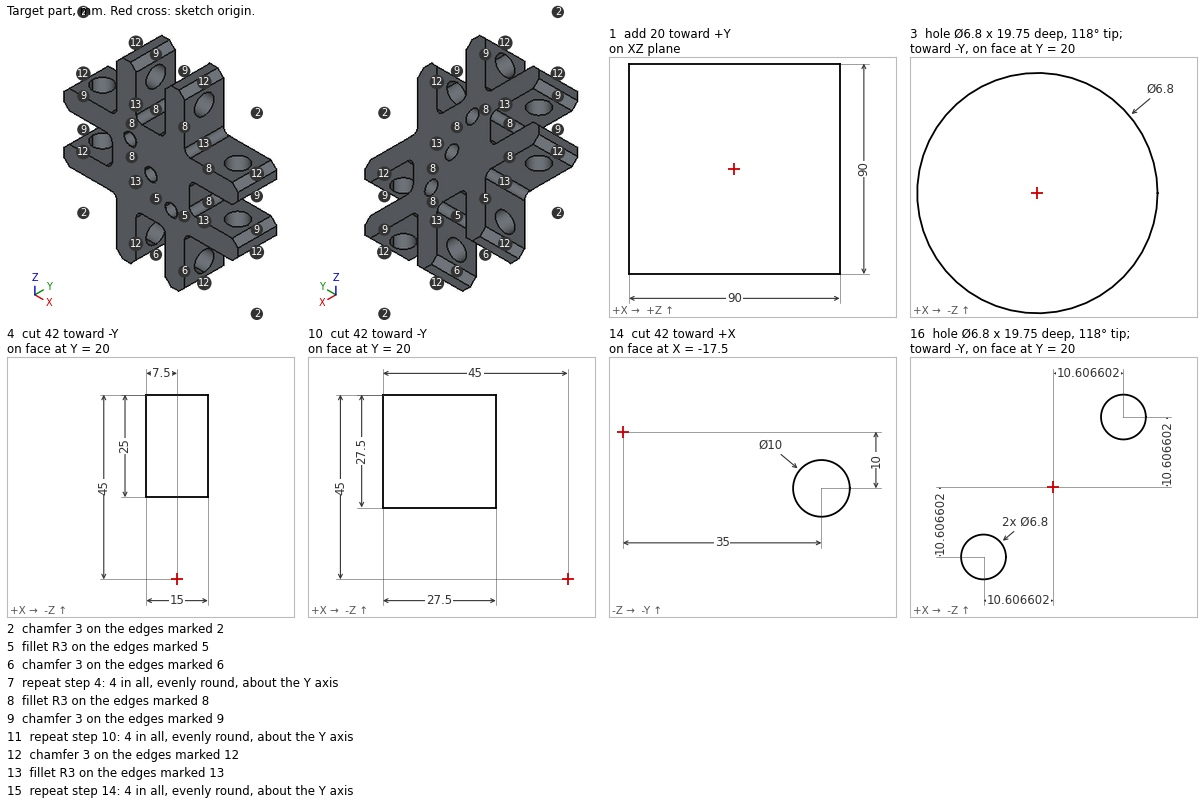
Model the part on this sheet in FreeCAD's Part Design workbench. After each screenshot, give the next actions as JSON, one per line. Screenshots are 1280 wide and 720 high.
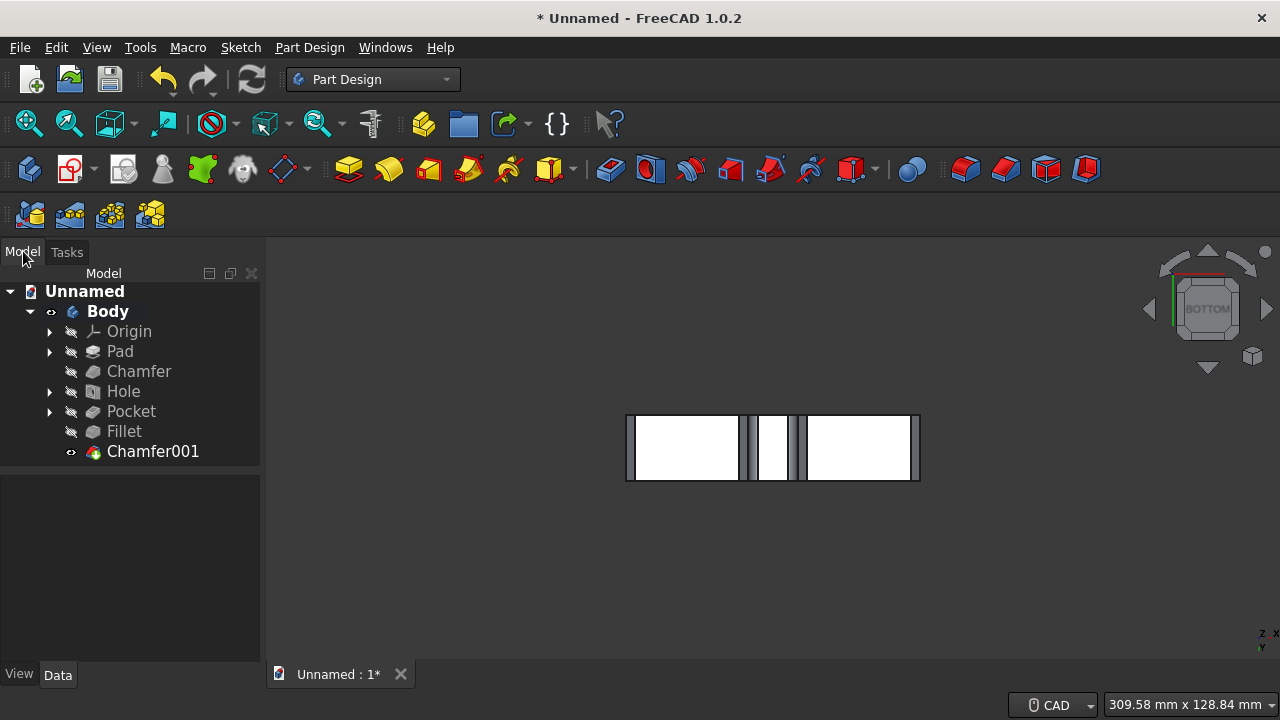
{"action": "left_click", "coordinate": [116, 412]}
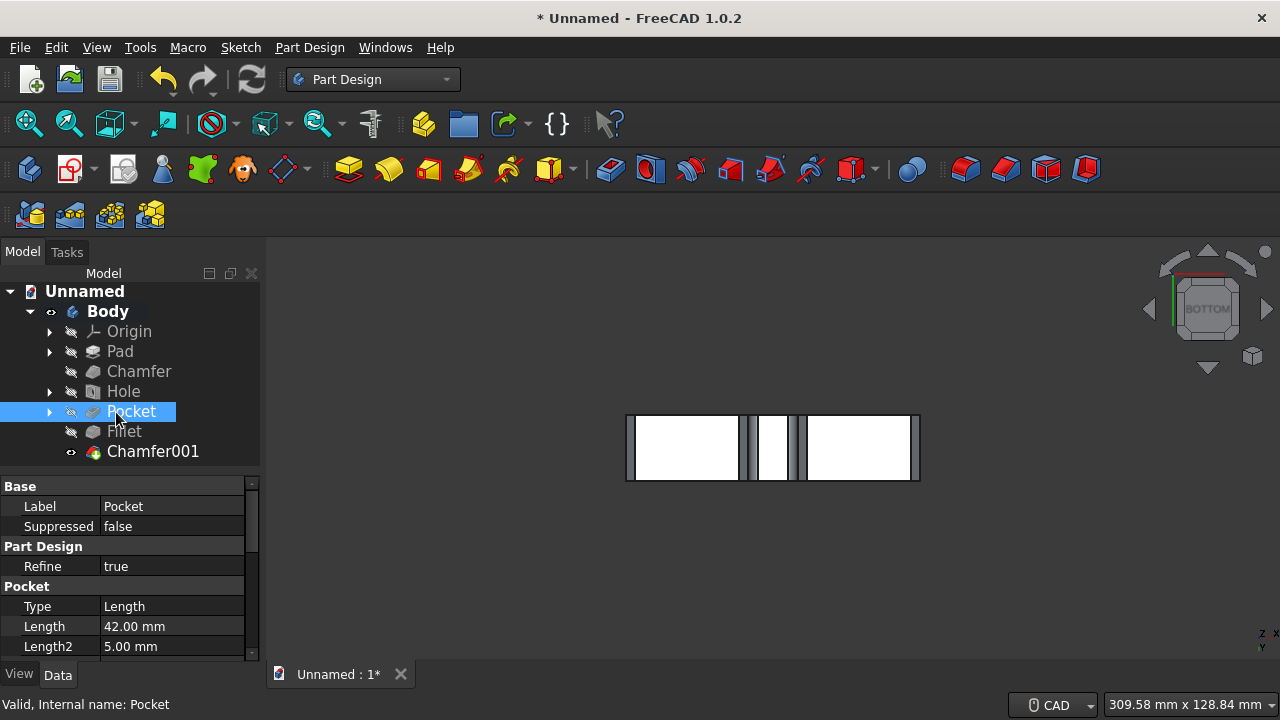
{"action": "left_click", "coordinate": [110, 214]}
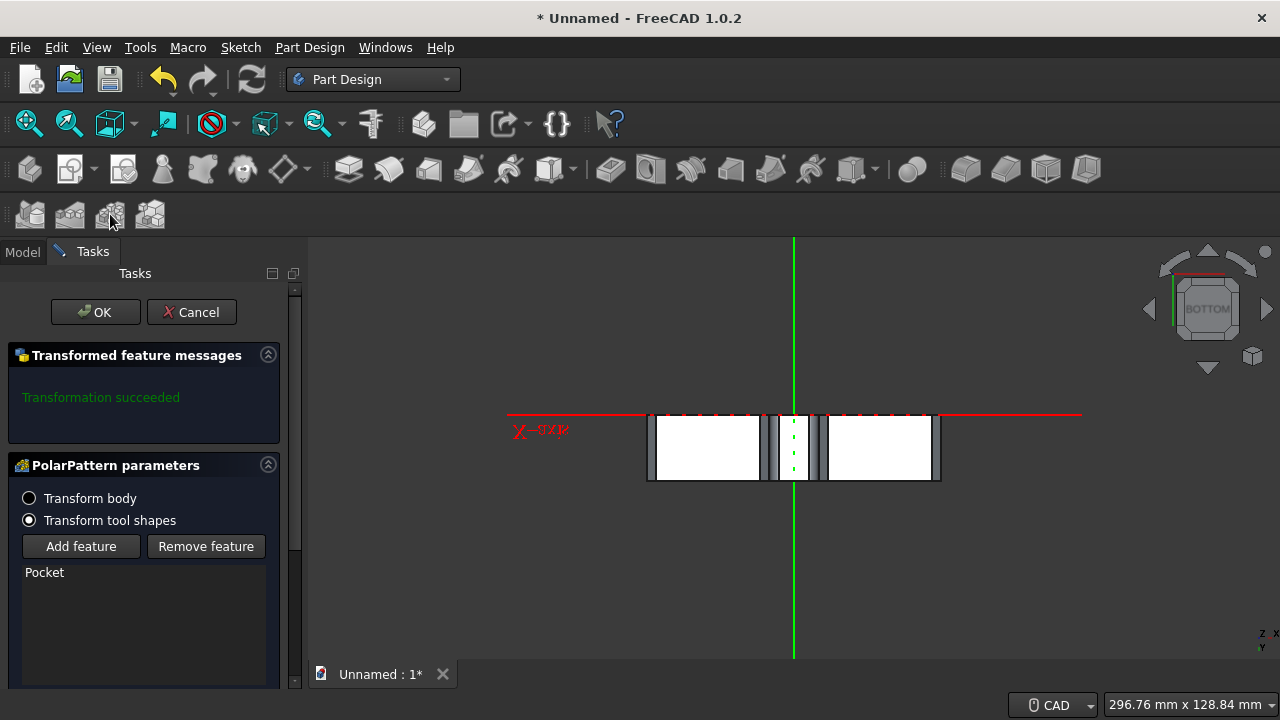
{"action": "scroll", "coordinate": [295, 486], "scroll_direction": "down", "scroll_amount": 2}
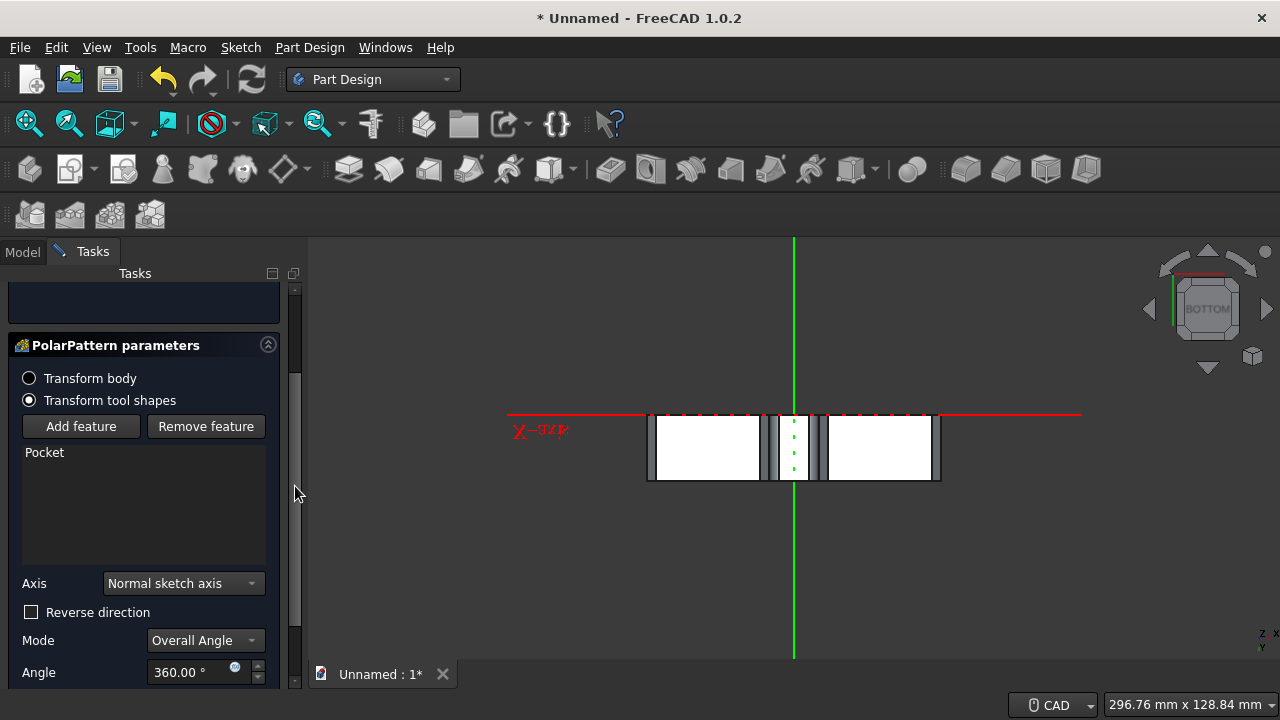
{"action": "left_click", "coordinate": [184, 584]}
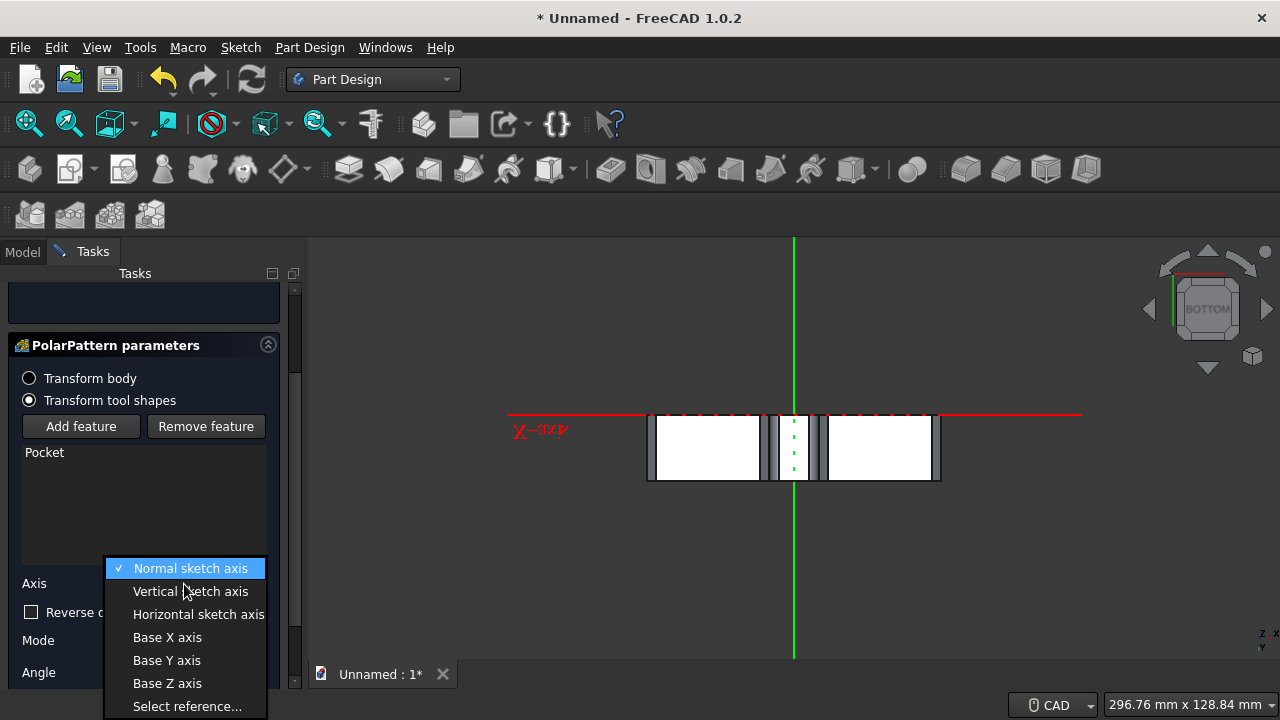
{"action": "left_click", "coordinate": [184, 660]}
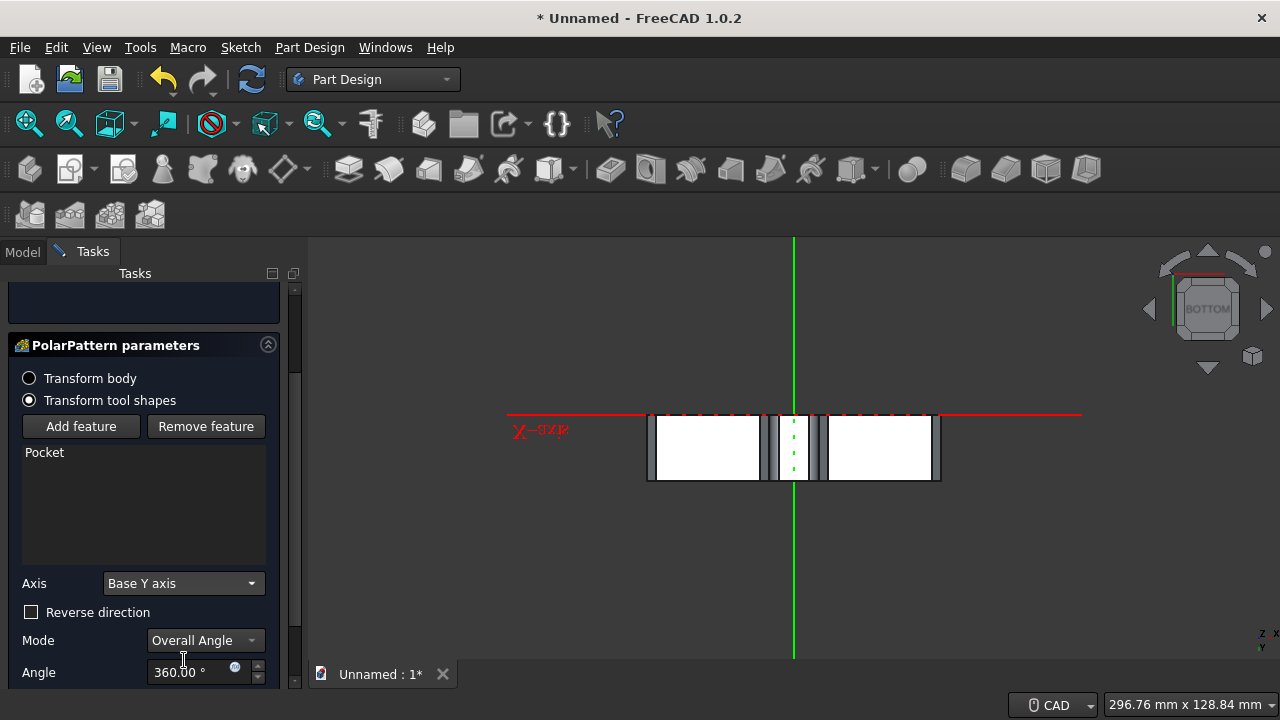
{"action": "scroll", "coordinate": [295, 486], "scroll_direction": "down", "scroll_amount": 2}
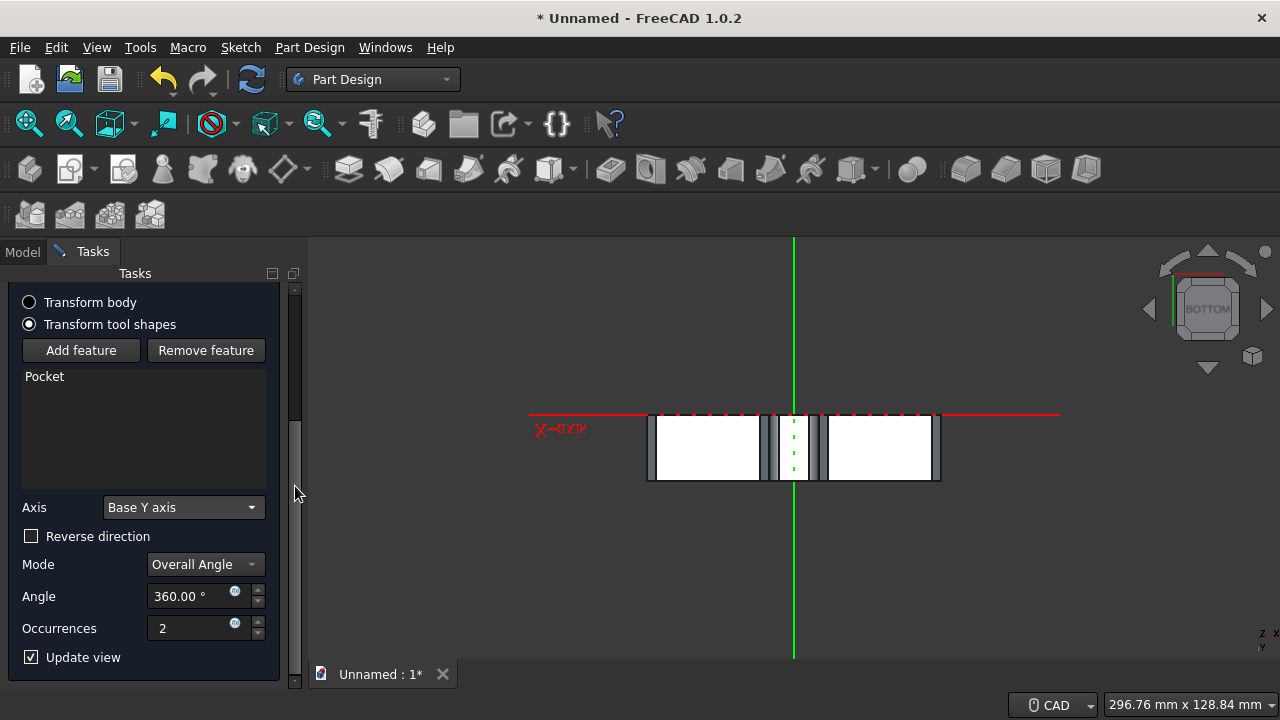
{"action": "triple_click", "coordinate": [198, 628]}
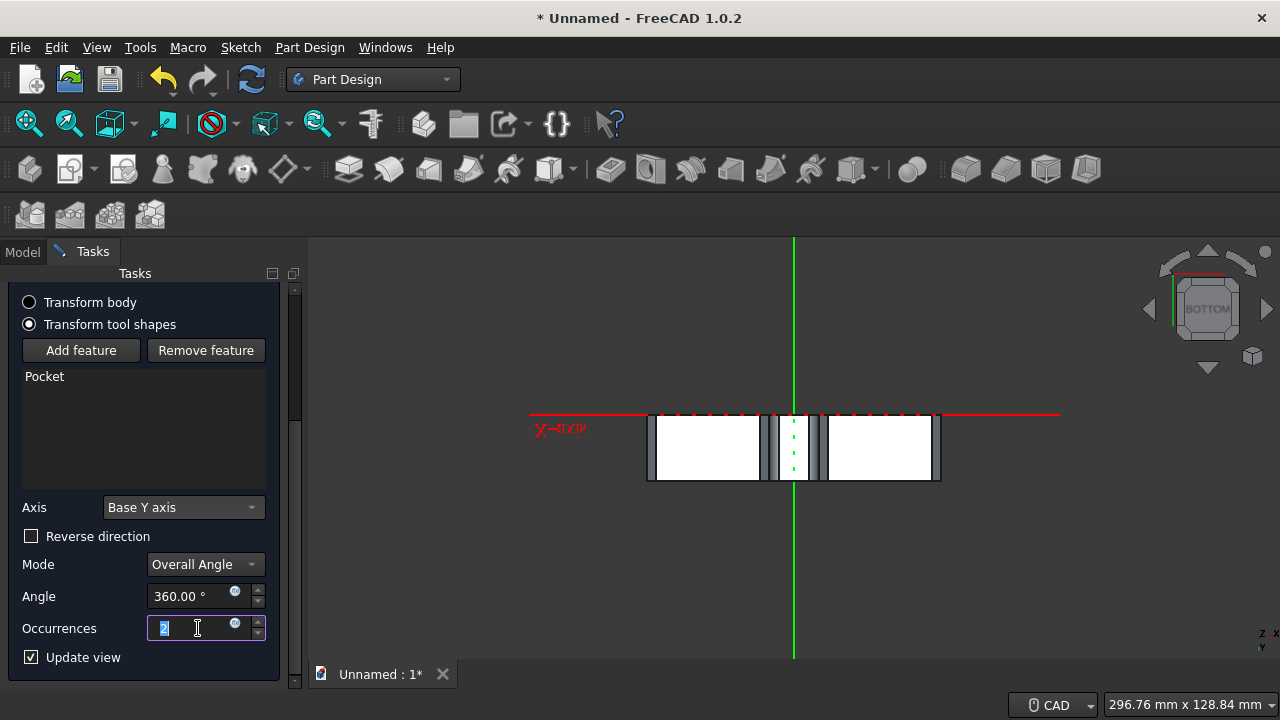
{"action": "type", "text": "4"}
{"action": "key", "text": "Tab"}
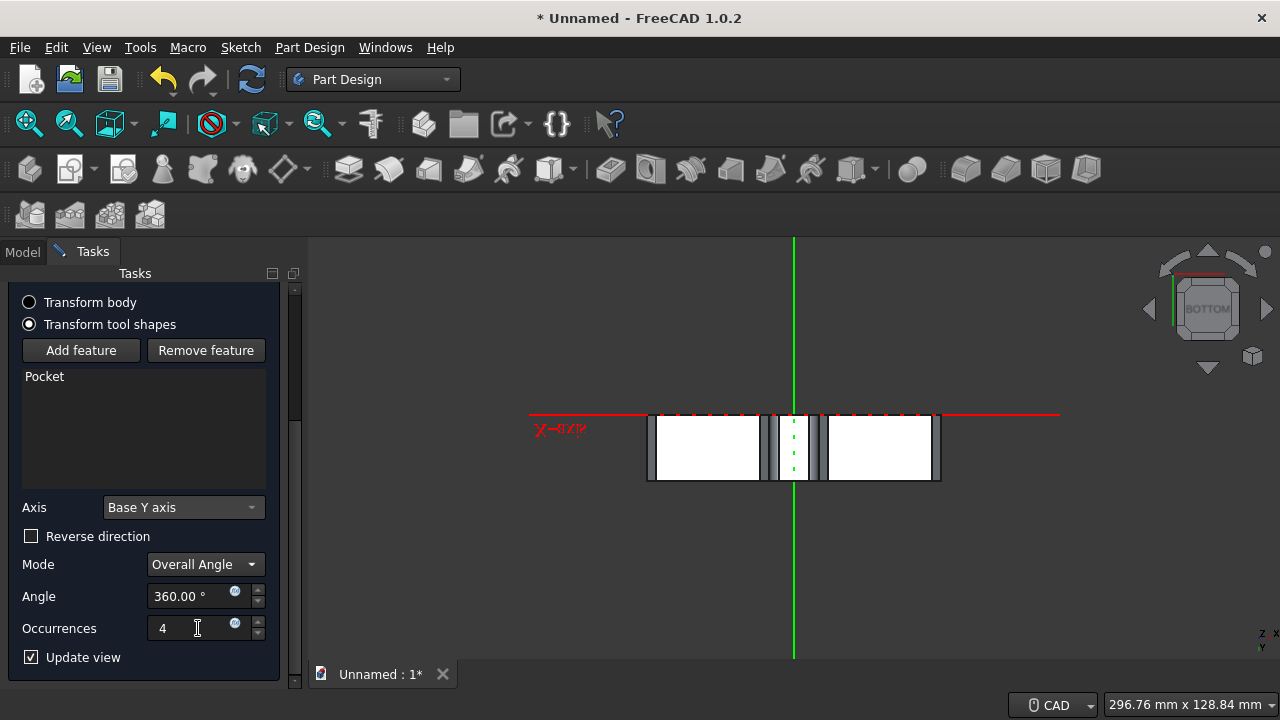
{"action": "scroll", "coordinate": [295, 486], "scroll_direction": "up", "scroll_amount": 5}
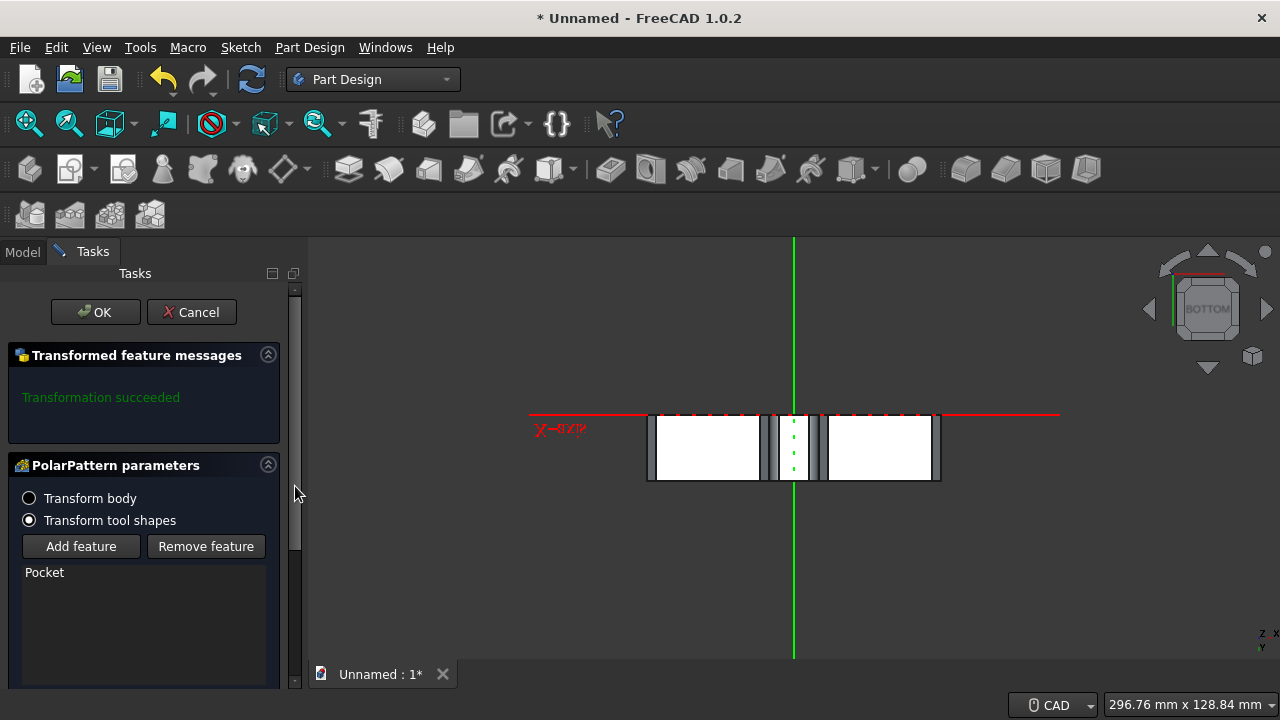
{"action": "left_click", "coordinate": [96, 312]}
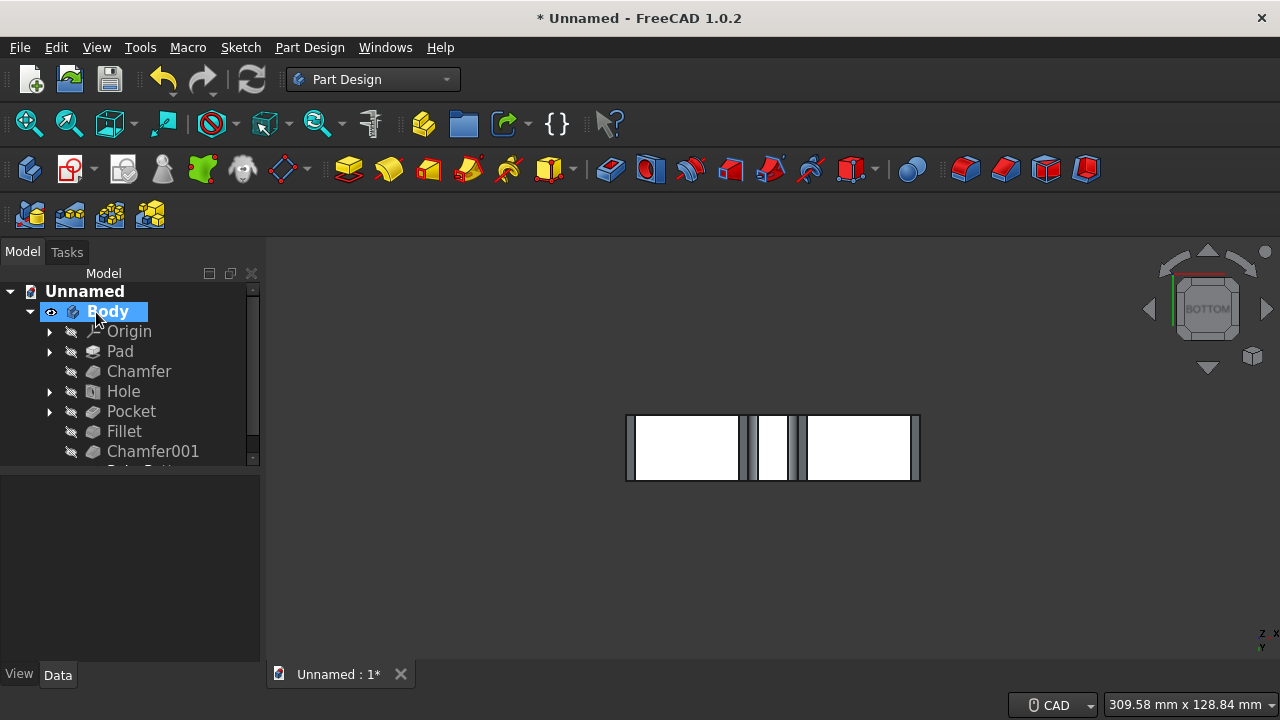
{"action": "left_click", "coordinate": [30, 124]}